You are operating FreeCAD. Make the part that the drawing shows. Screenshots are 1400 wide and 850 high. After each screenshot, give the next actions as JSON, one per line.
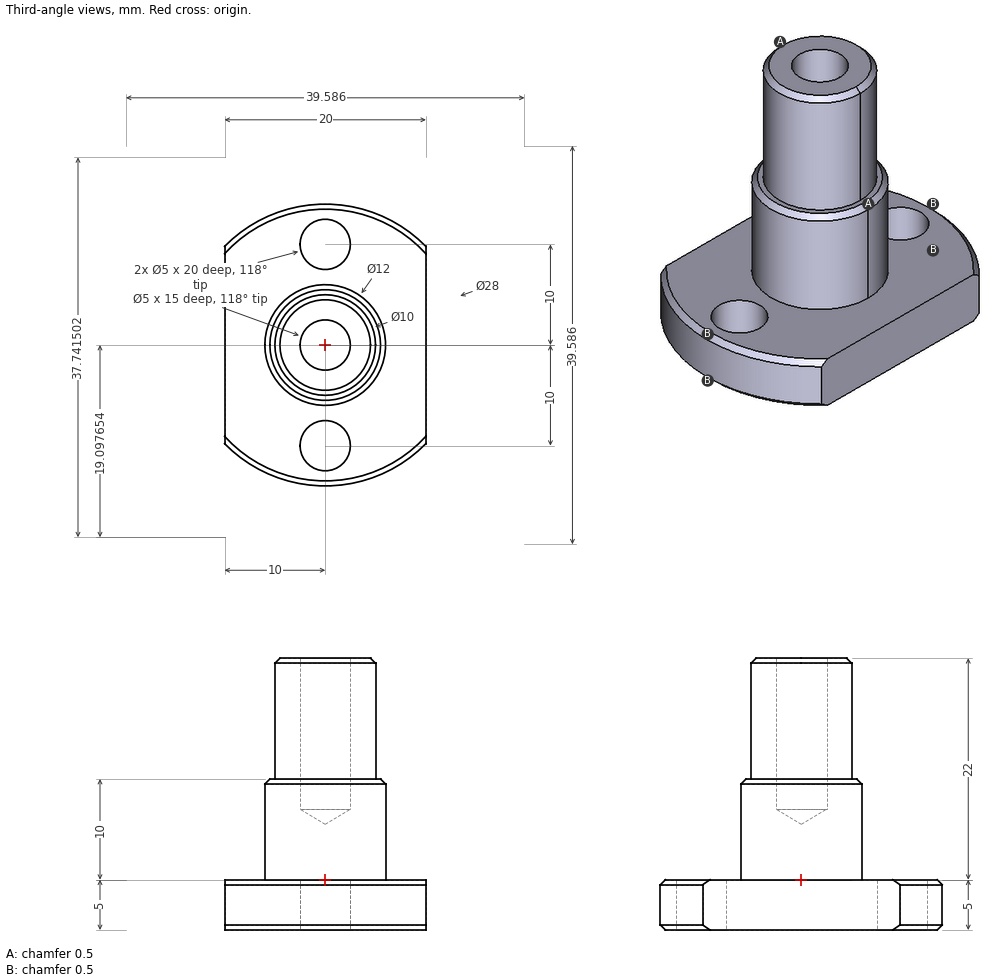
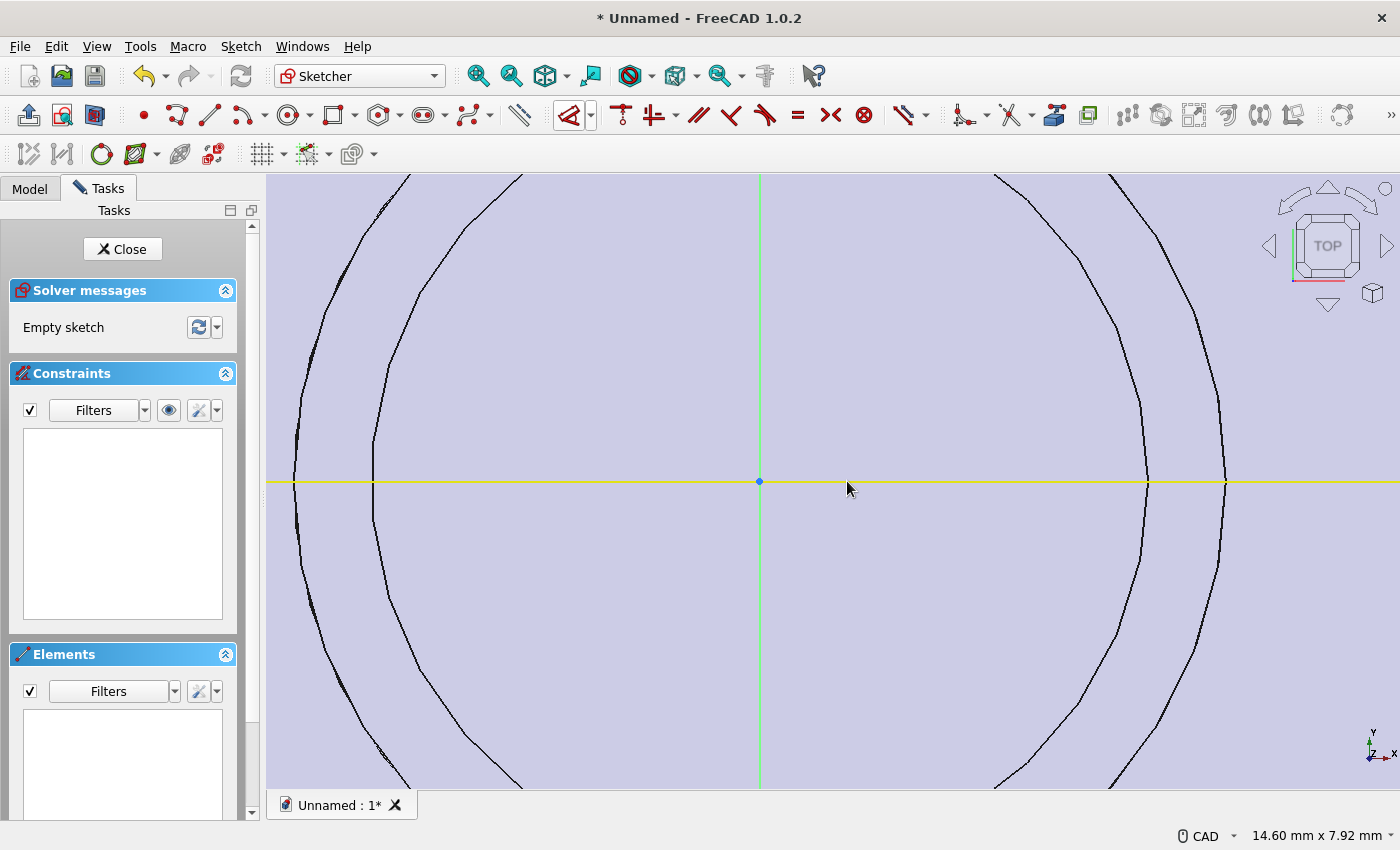
{"action": "left_click", "coordinate": [288, 116]}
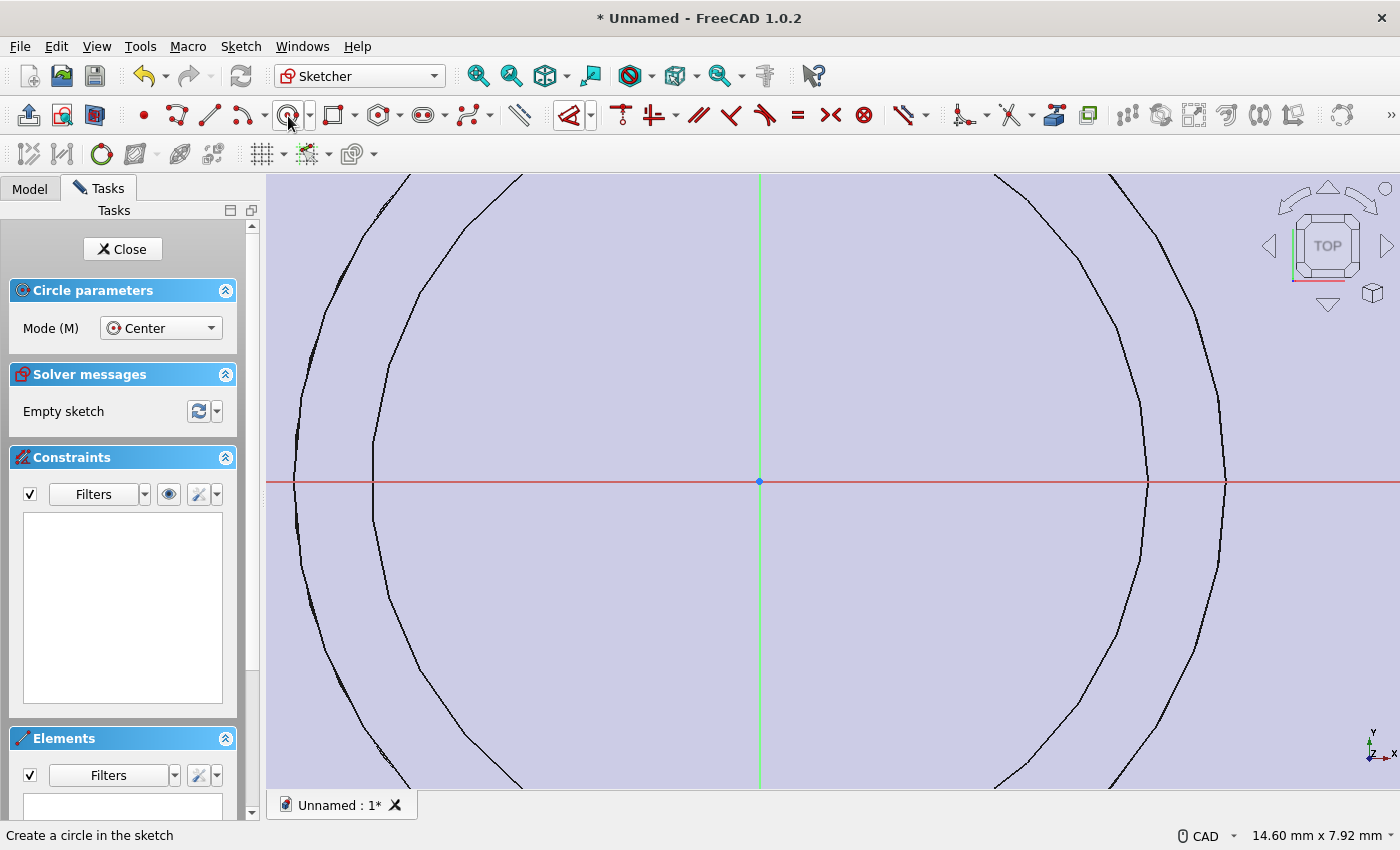
{"action": "left_click", "coordinate": [760, 481]}
{"action": "mouse_move", "coordinate": [897, 344]}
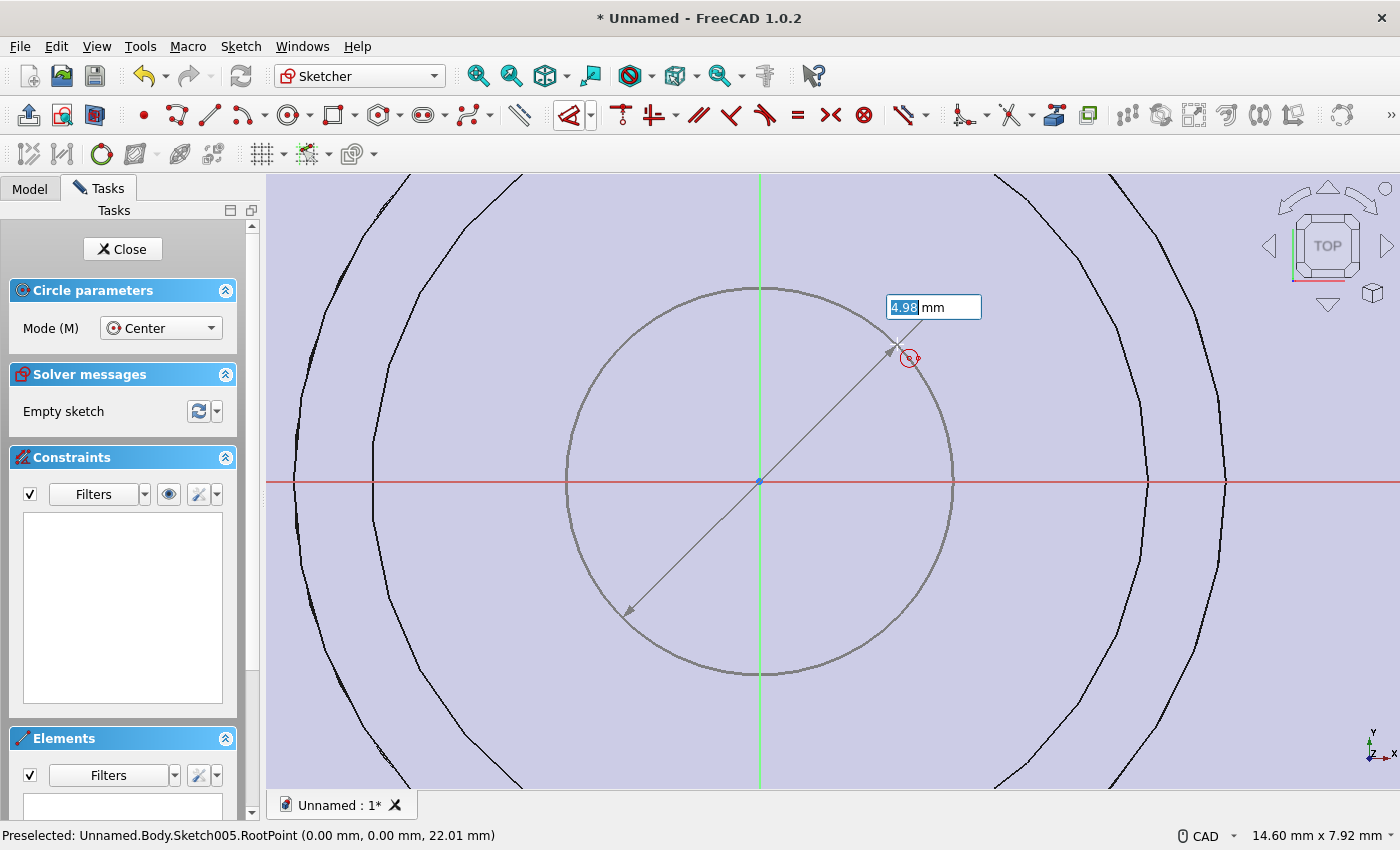
{"action": "type", "text": "5"}
{"action": "key", "text": "Return"}
{"action": "key", "text": "Escape"}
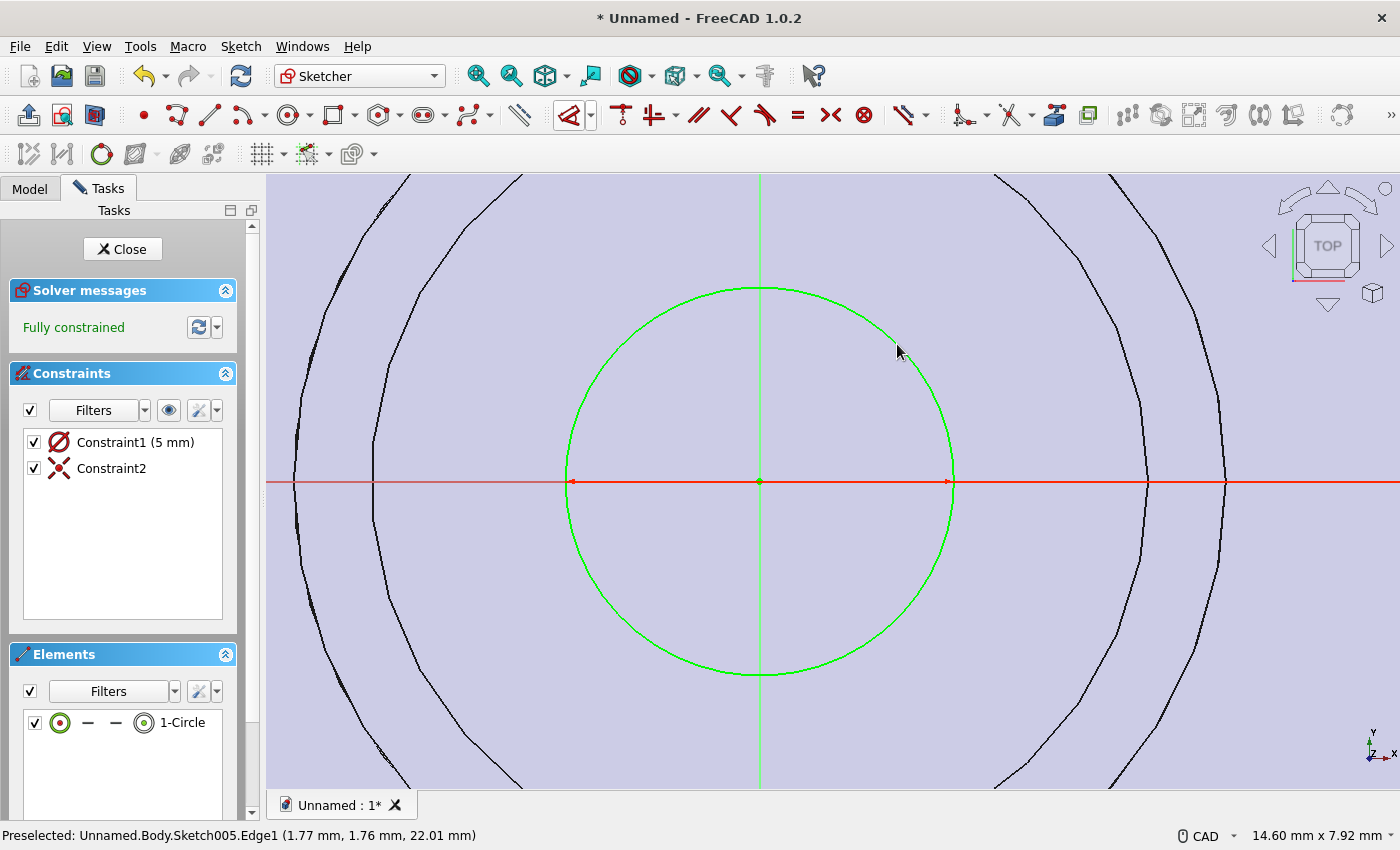
{"action": "left_click", "coordinate": [123, 249]}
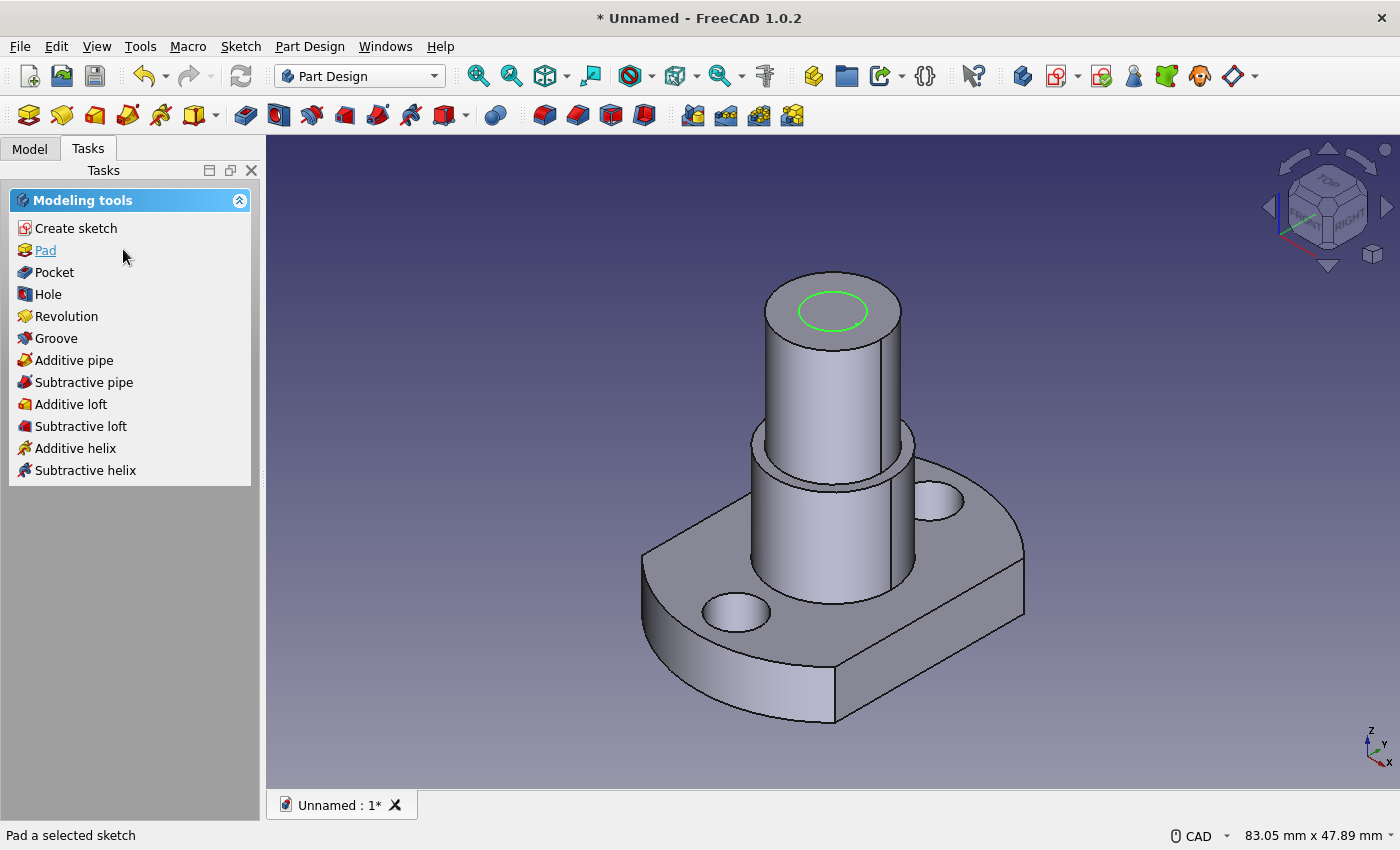
{"action": "left_click", "coordinate": [279, 116]}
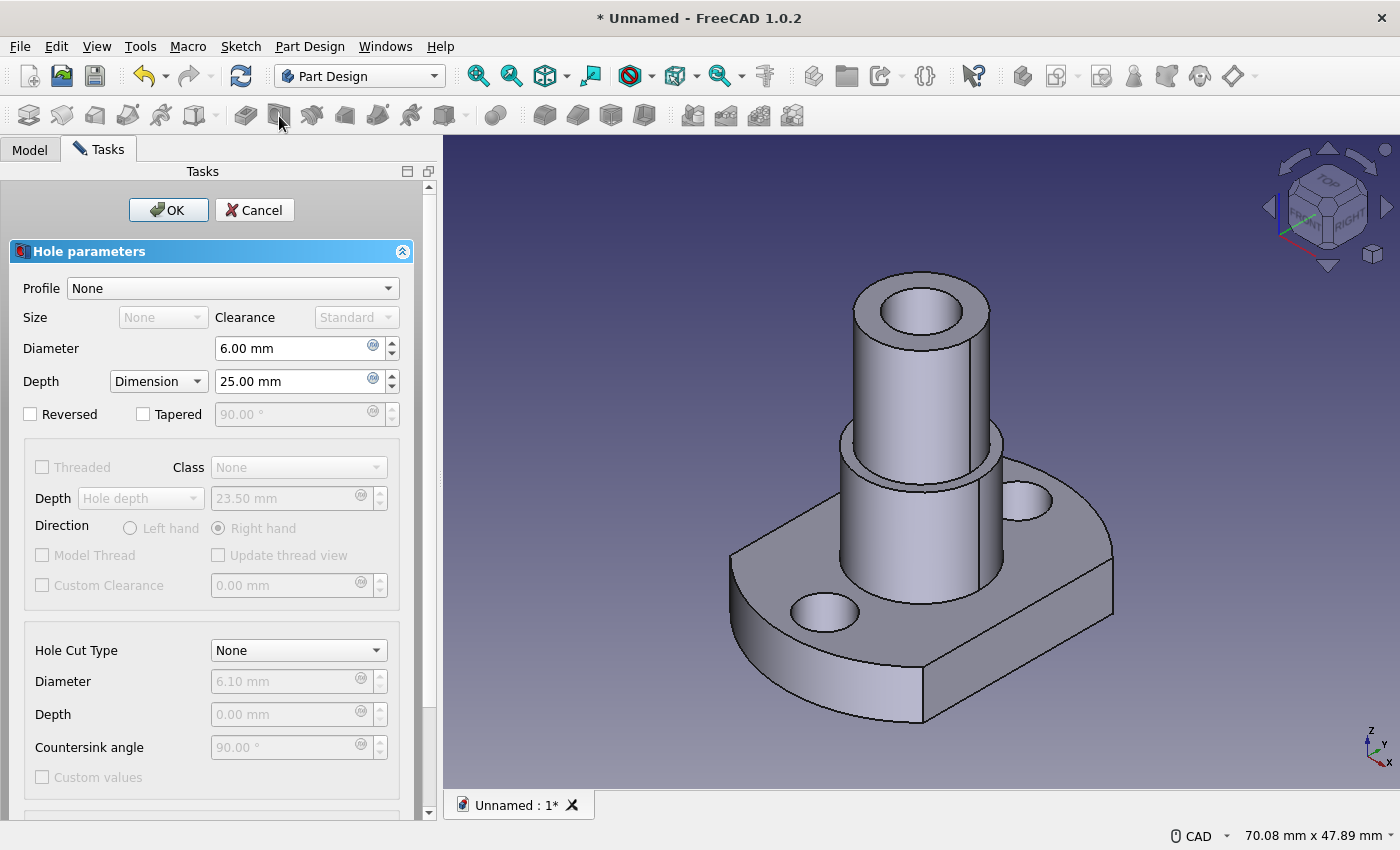
{"action": "triple_click", "coordinate": [300, 348]}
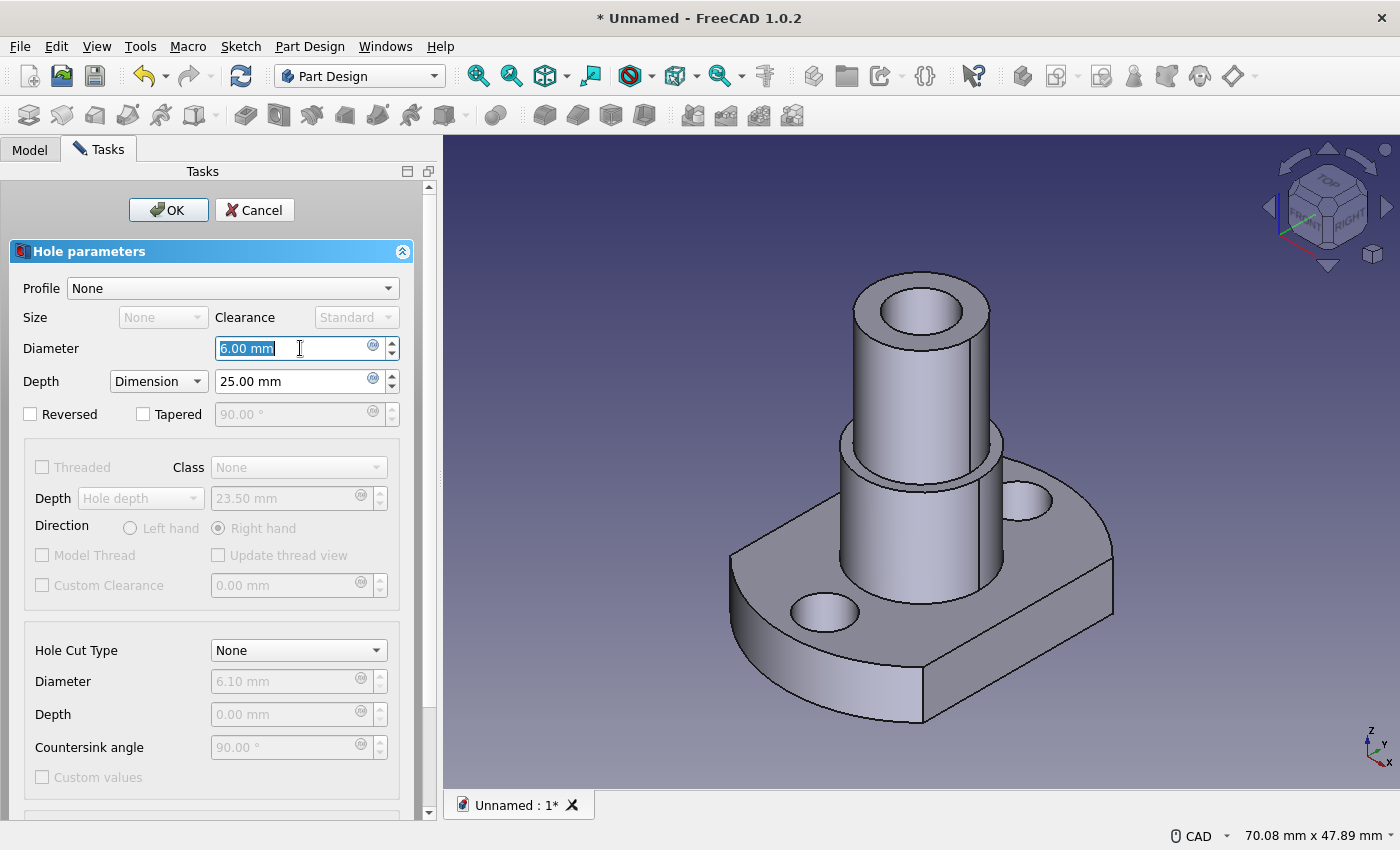
{"action": "type", "text": "5"}
{"action": "key", "text": "Tab"}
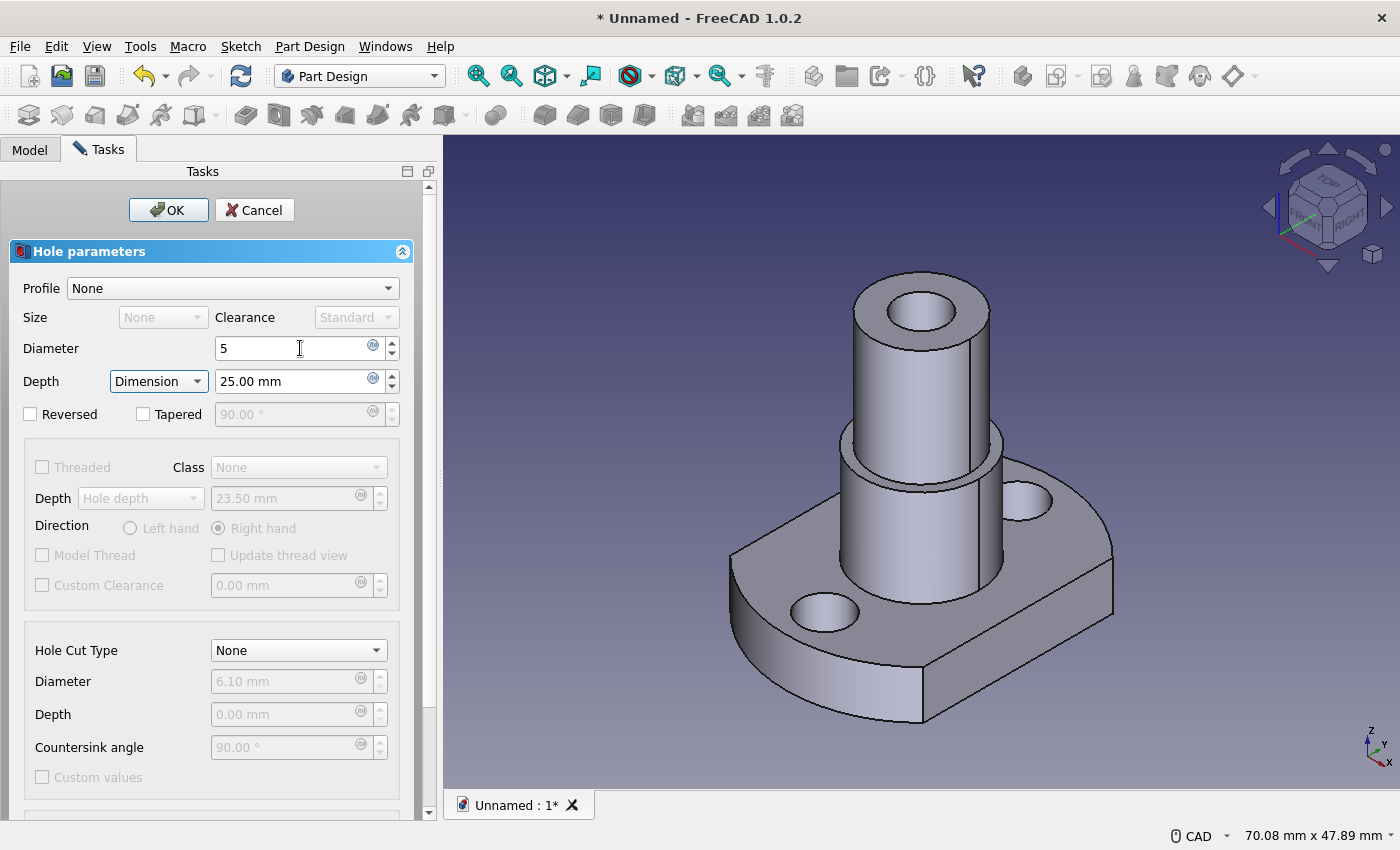
{"action": "triple_click", "coordinate": [300, 382]}